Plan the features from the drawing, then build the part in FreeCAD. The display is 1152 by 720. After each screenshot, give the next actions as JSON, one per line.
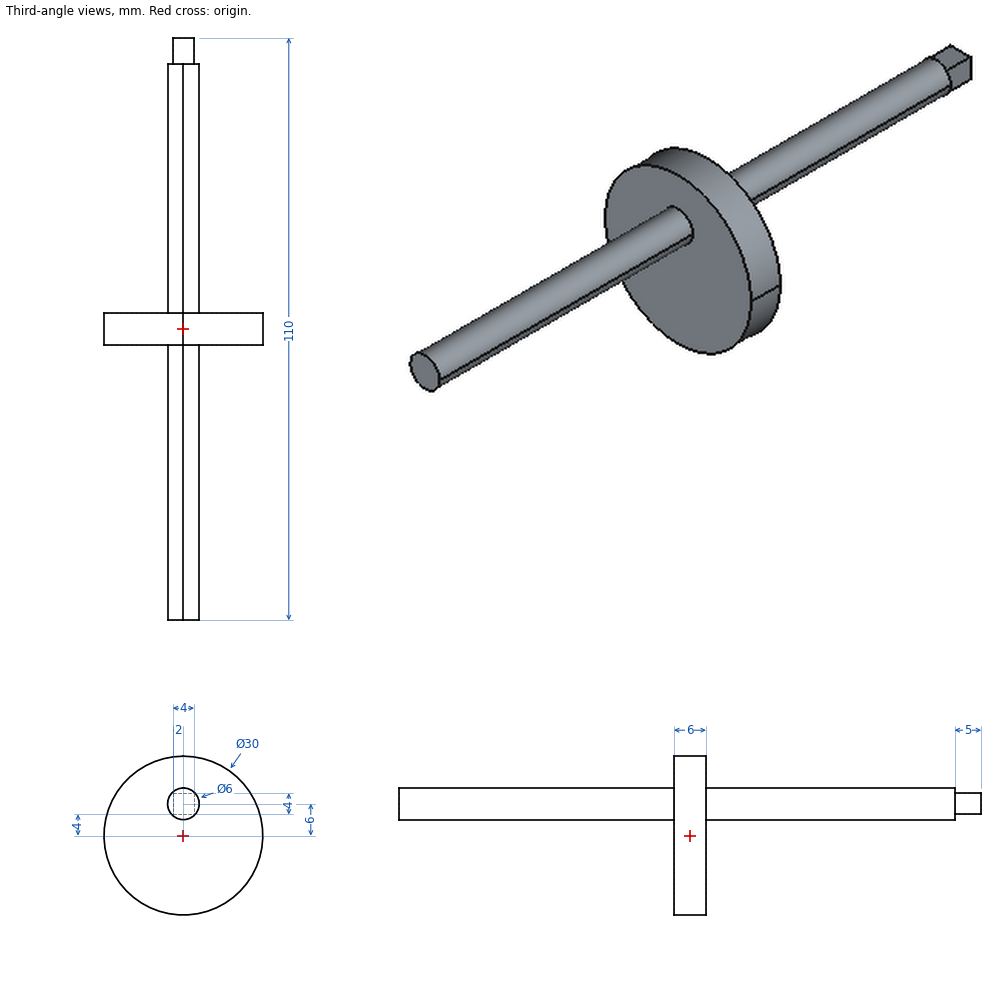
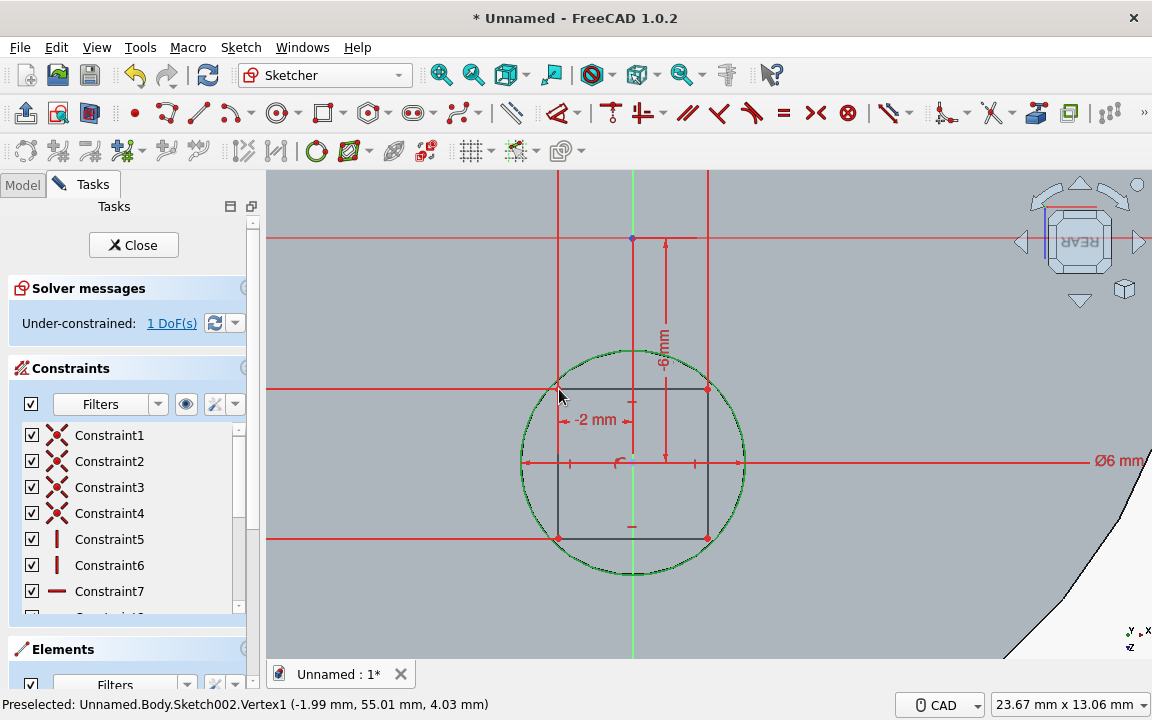
{"action": "left_click", "coordinate": [558, 389]}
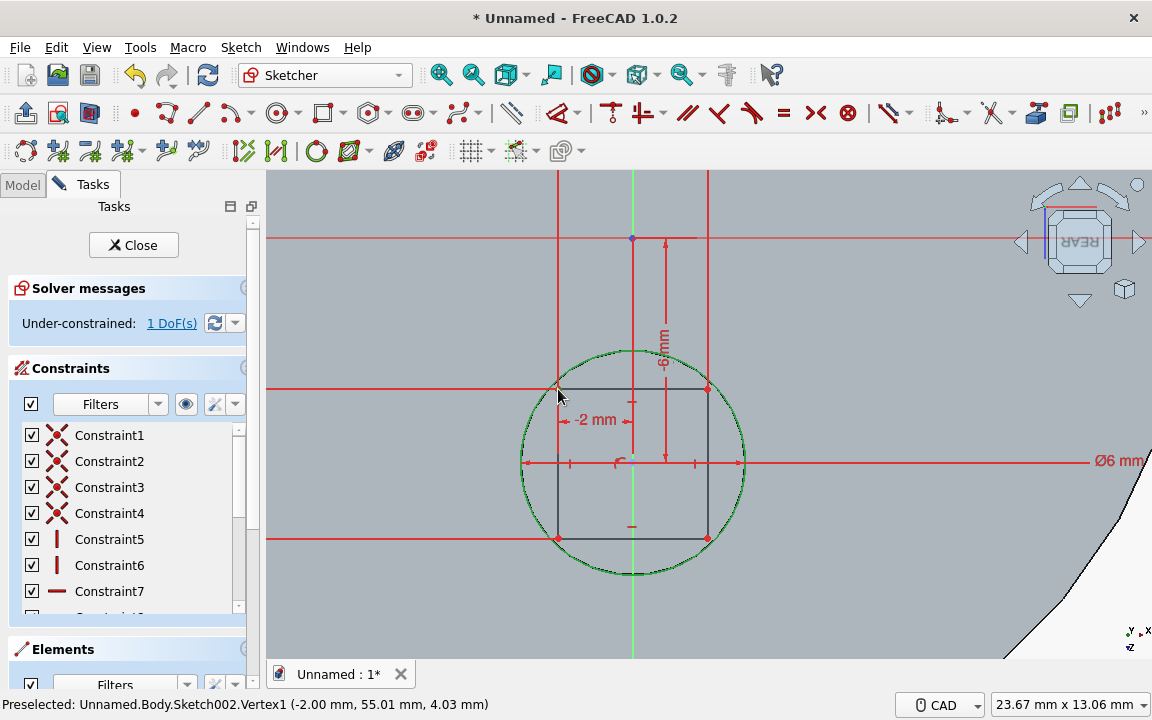
{"action": "key", "text": "i"}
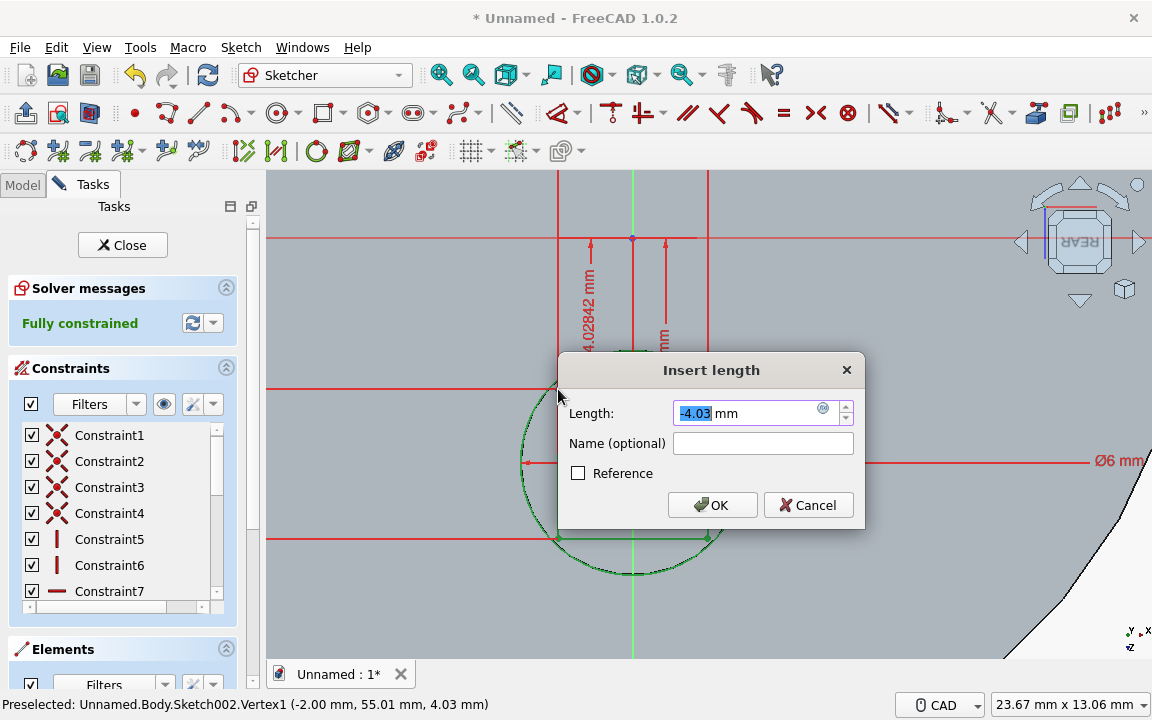
{"action": "type", "text": "-4"}
{"action": "key", "text": "Return"}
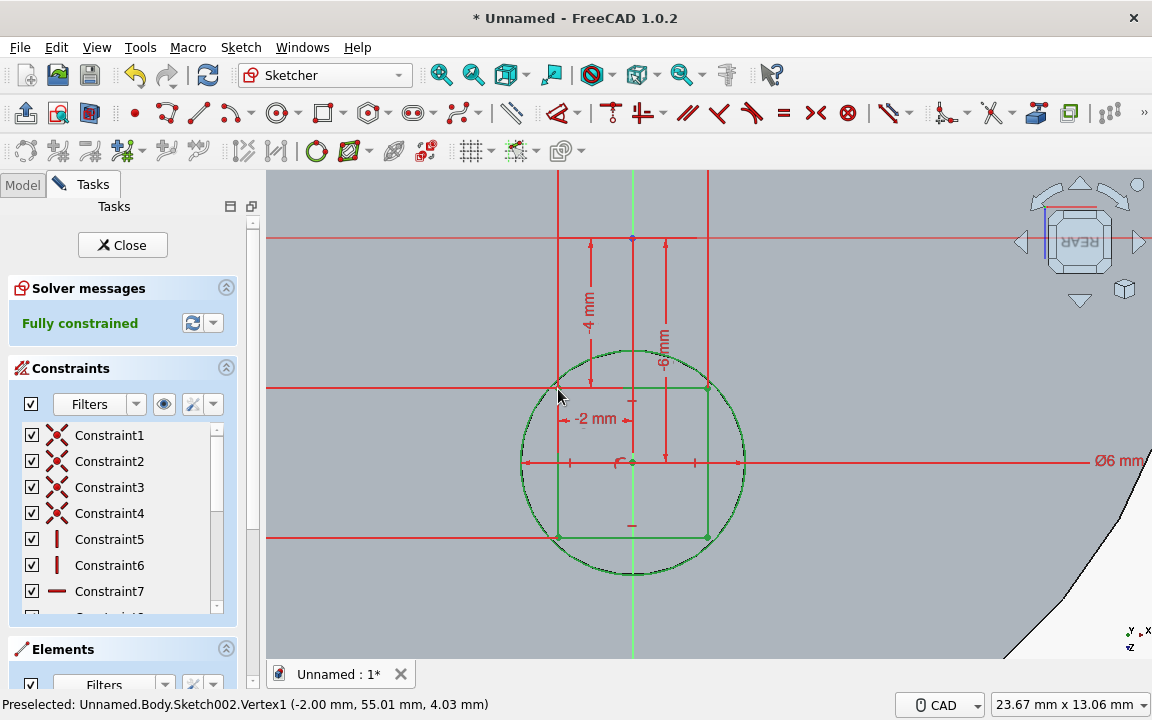
{"action": "left_click", "coordinate": [123, 245]}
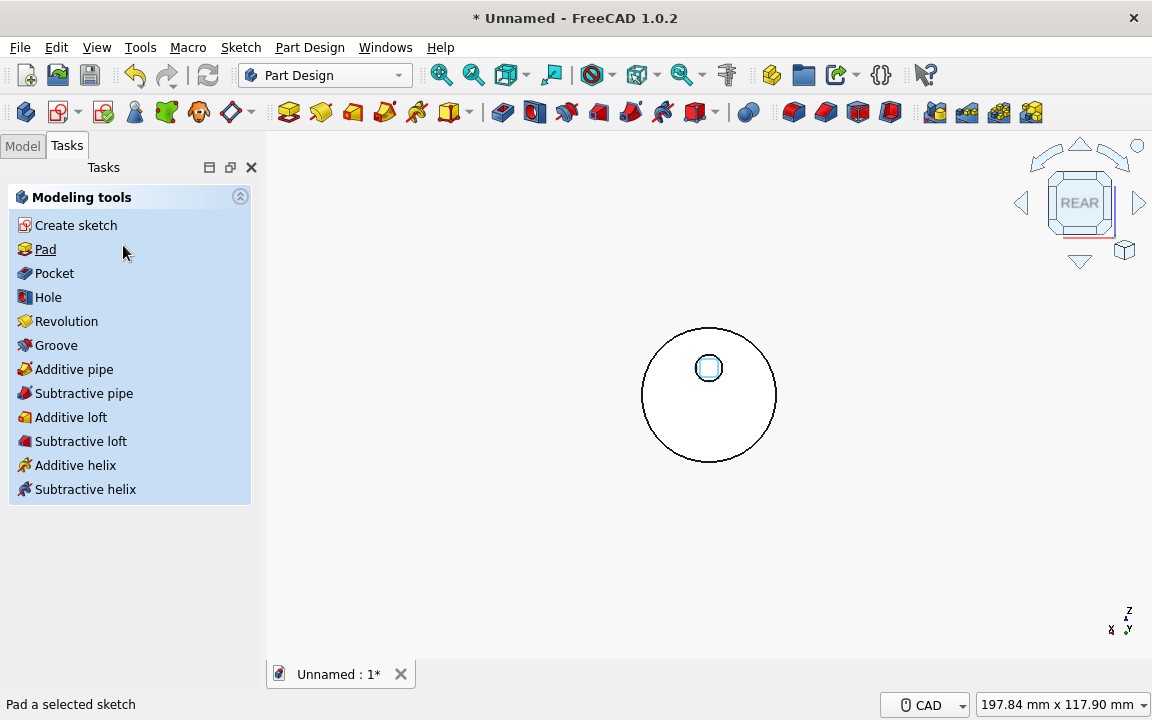
{"action": "left_click", "coordinate": [504, 112]}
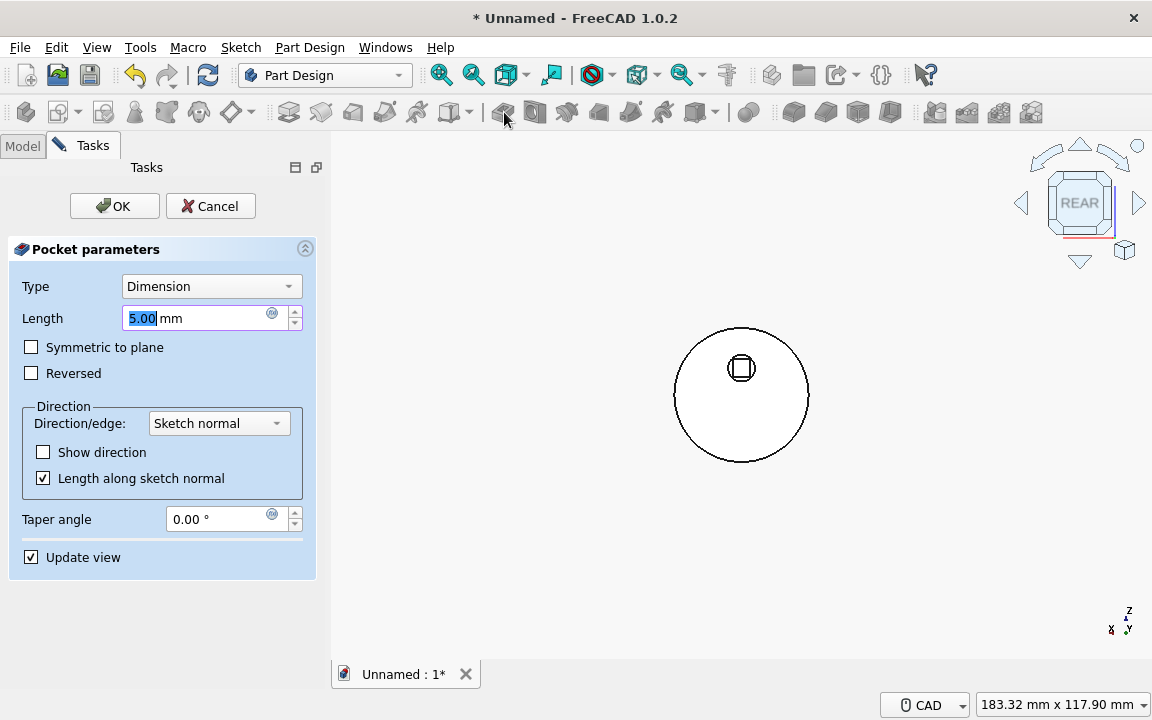
{"action": "type", "text": "5"}
{"action": "key", "text": "Tab"}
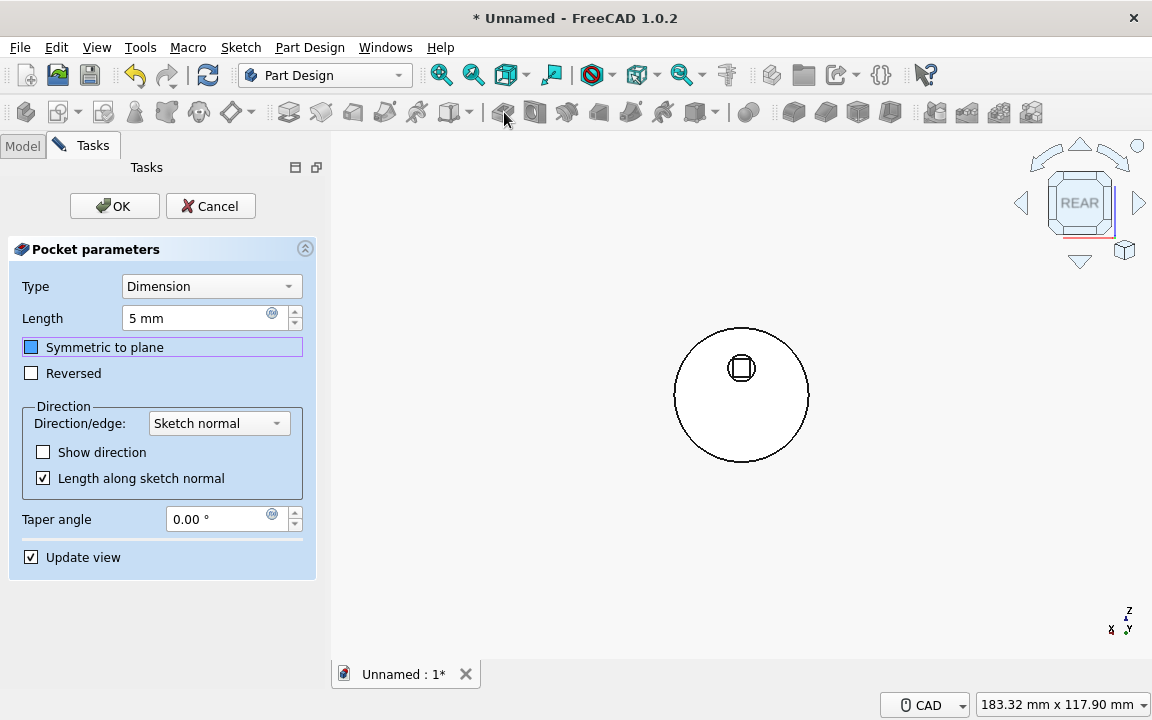
{"action": "left_click", "coordinate": [115, 206]}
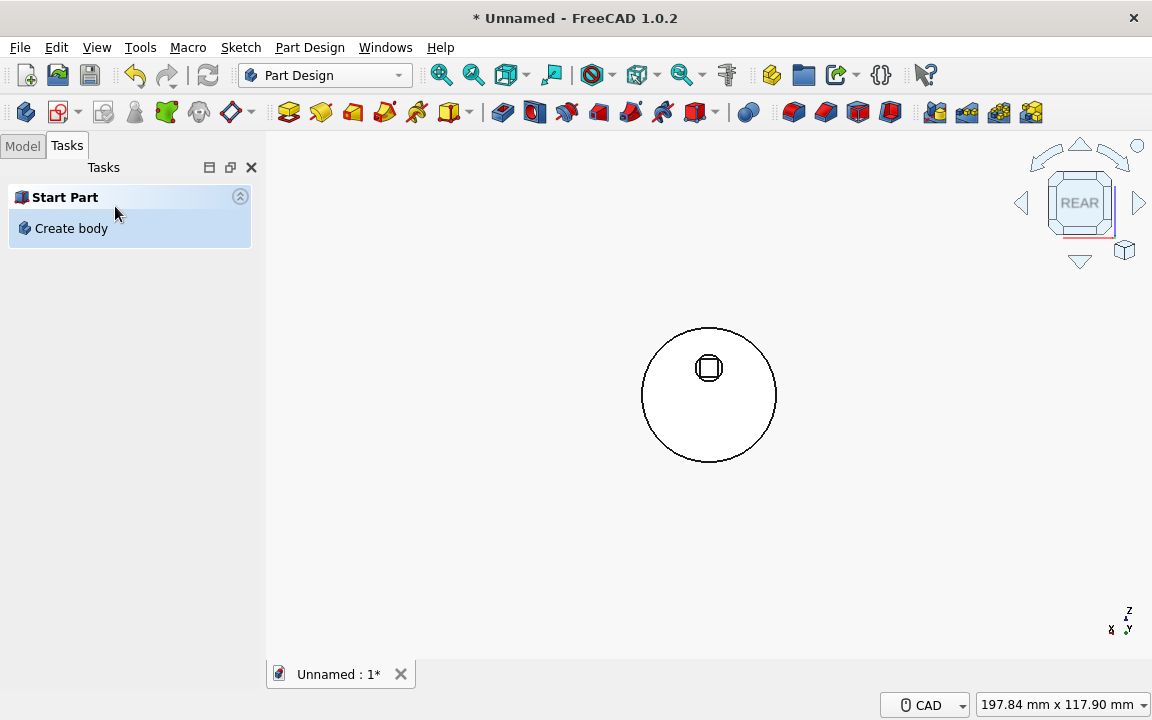
{"action": "key", "text": "0"}